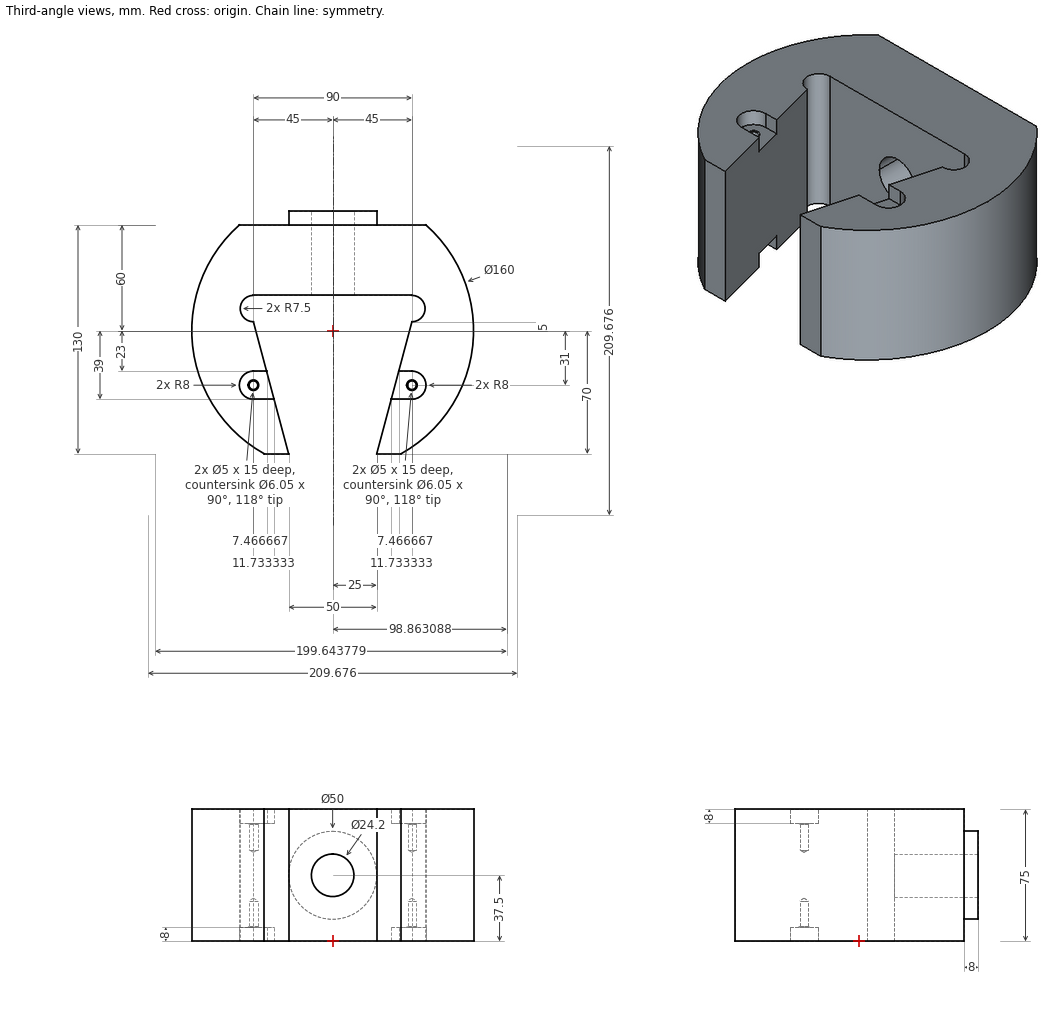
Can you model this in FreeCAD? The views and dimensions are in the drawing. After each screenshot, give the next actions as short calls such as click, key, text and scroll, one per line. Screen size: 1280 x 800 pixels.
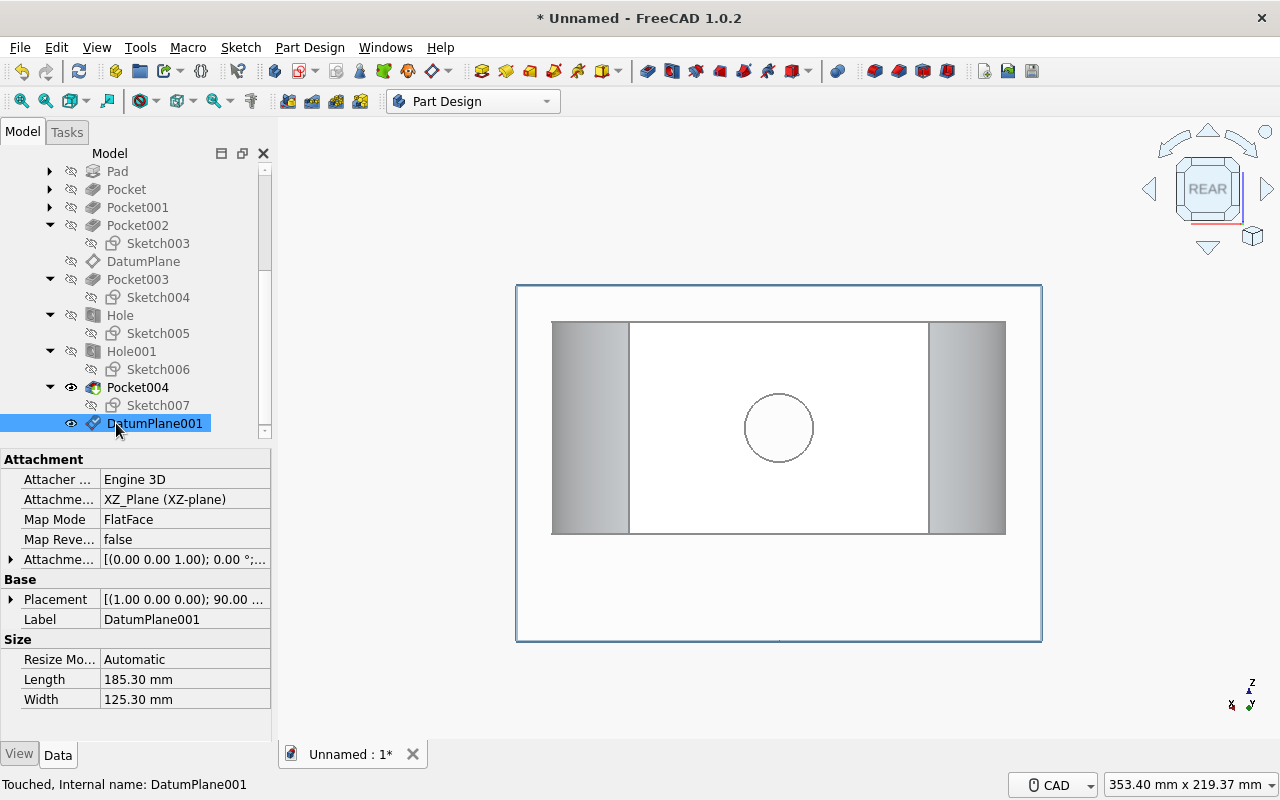
click(300, 72)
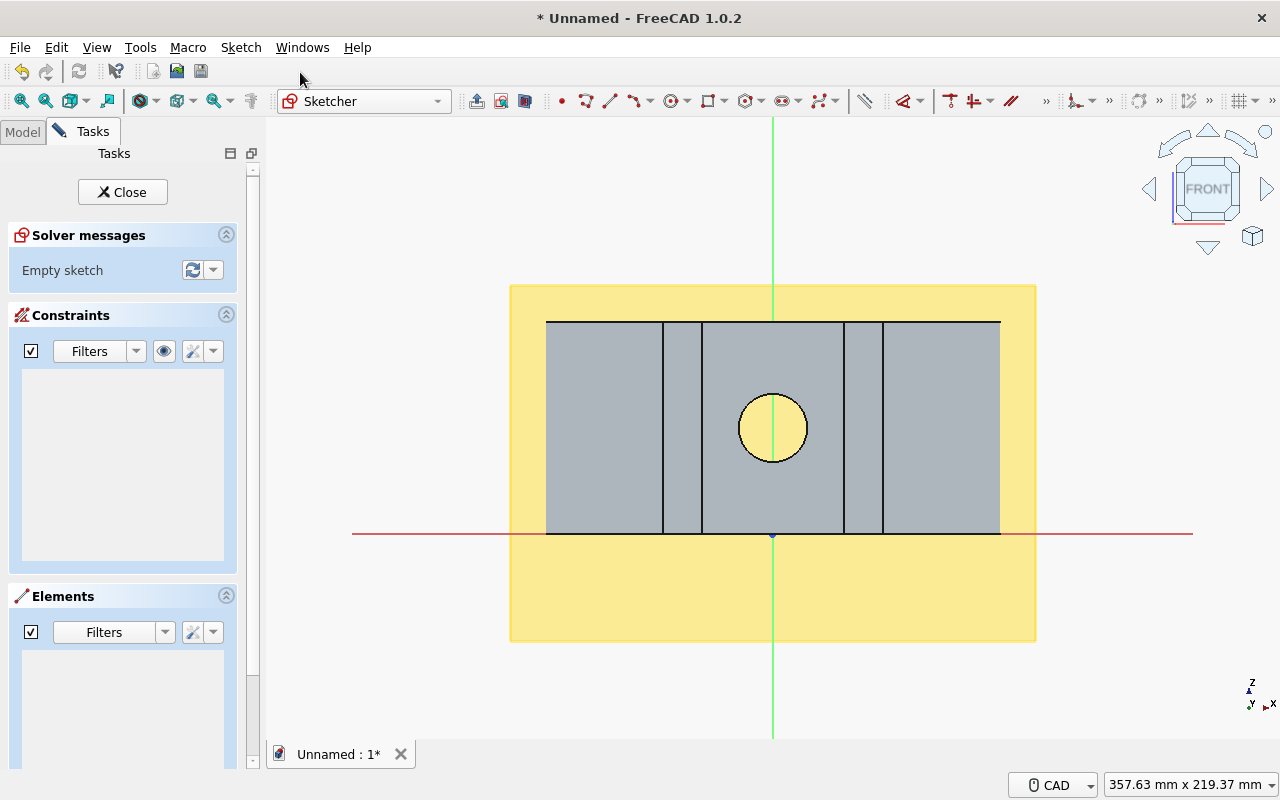
key(q)
key(s)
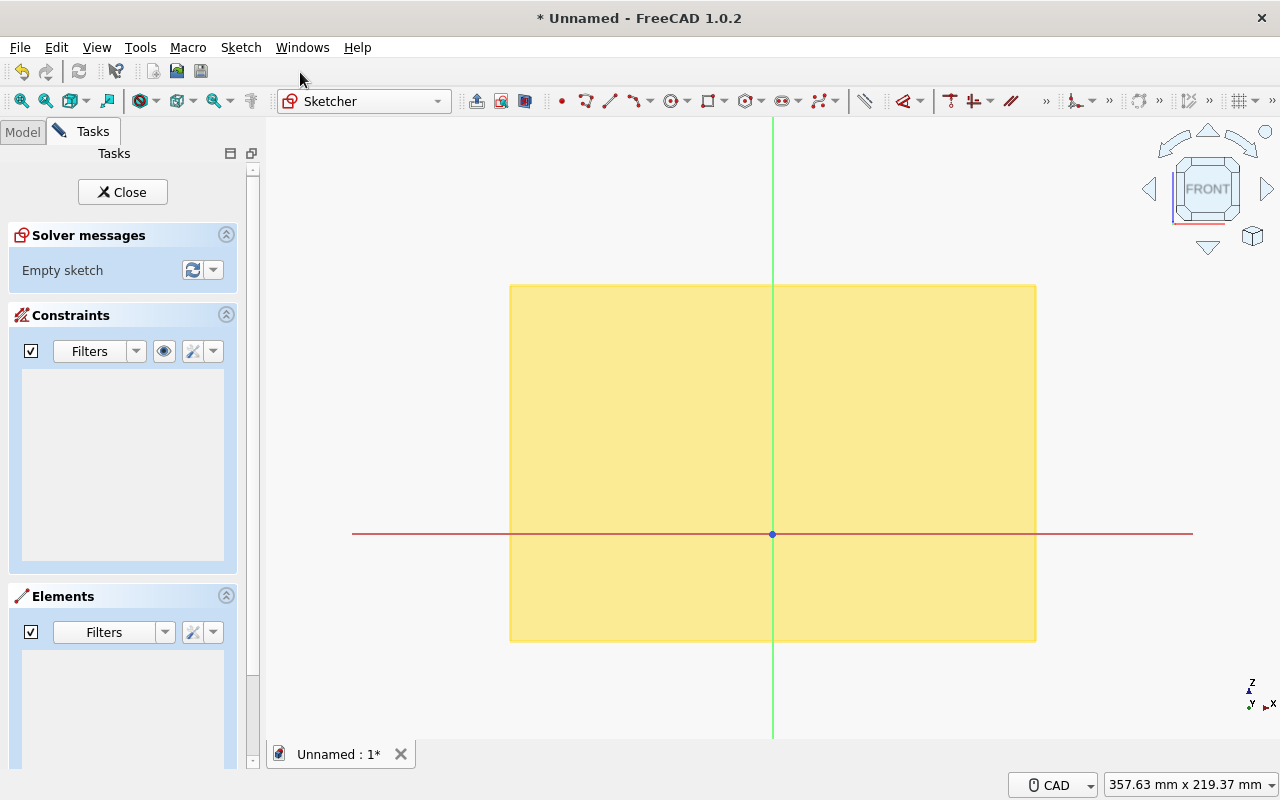
scroll(829, 460, up, 4)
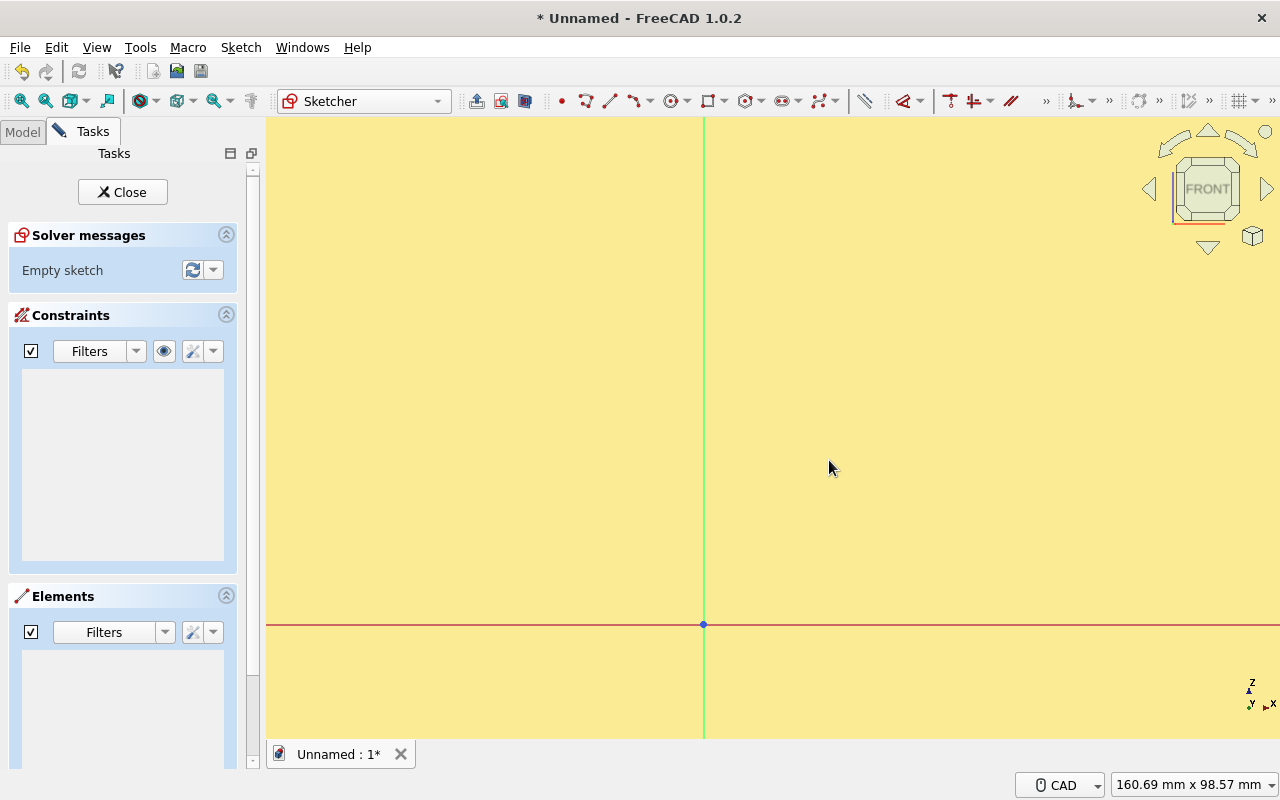
click(672, 102)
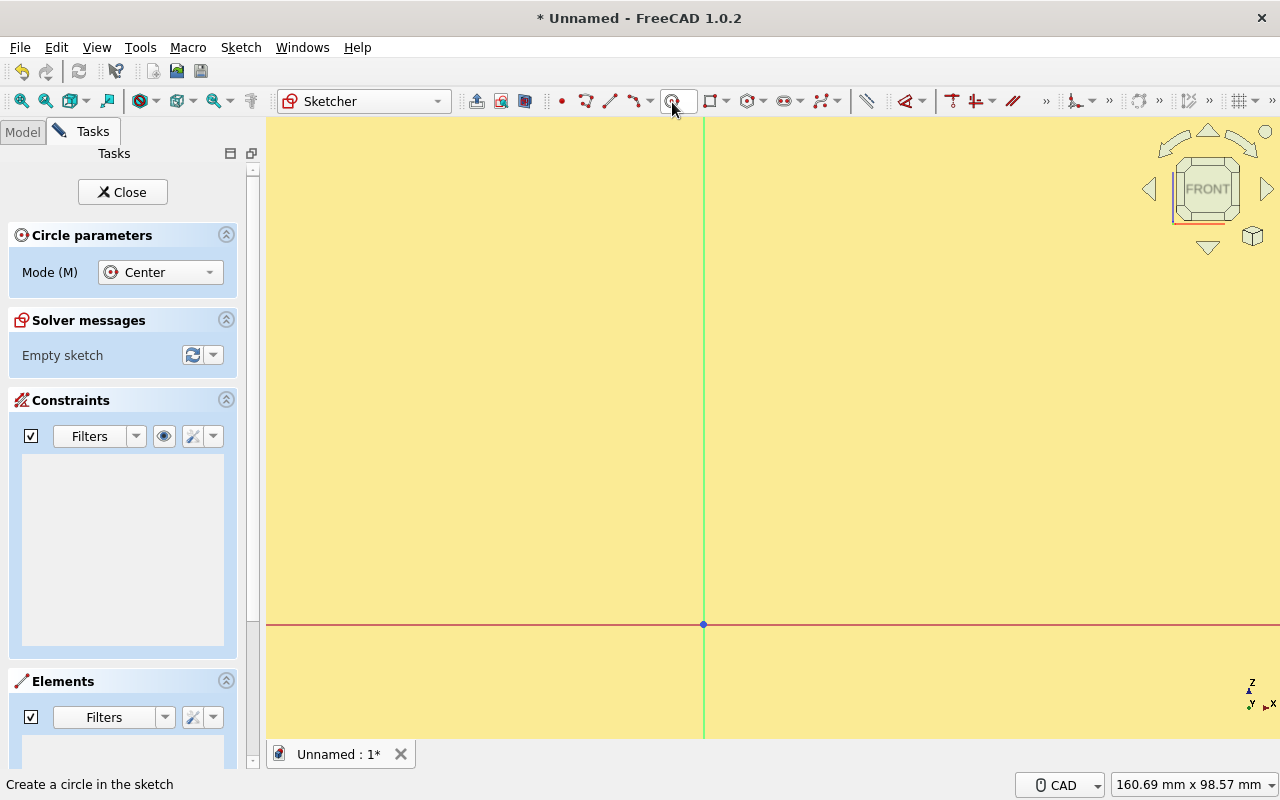
click(704, 388)
move(815, 277)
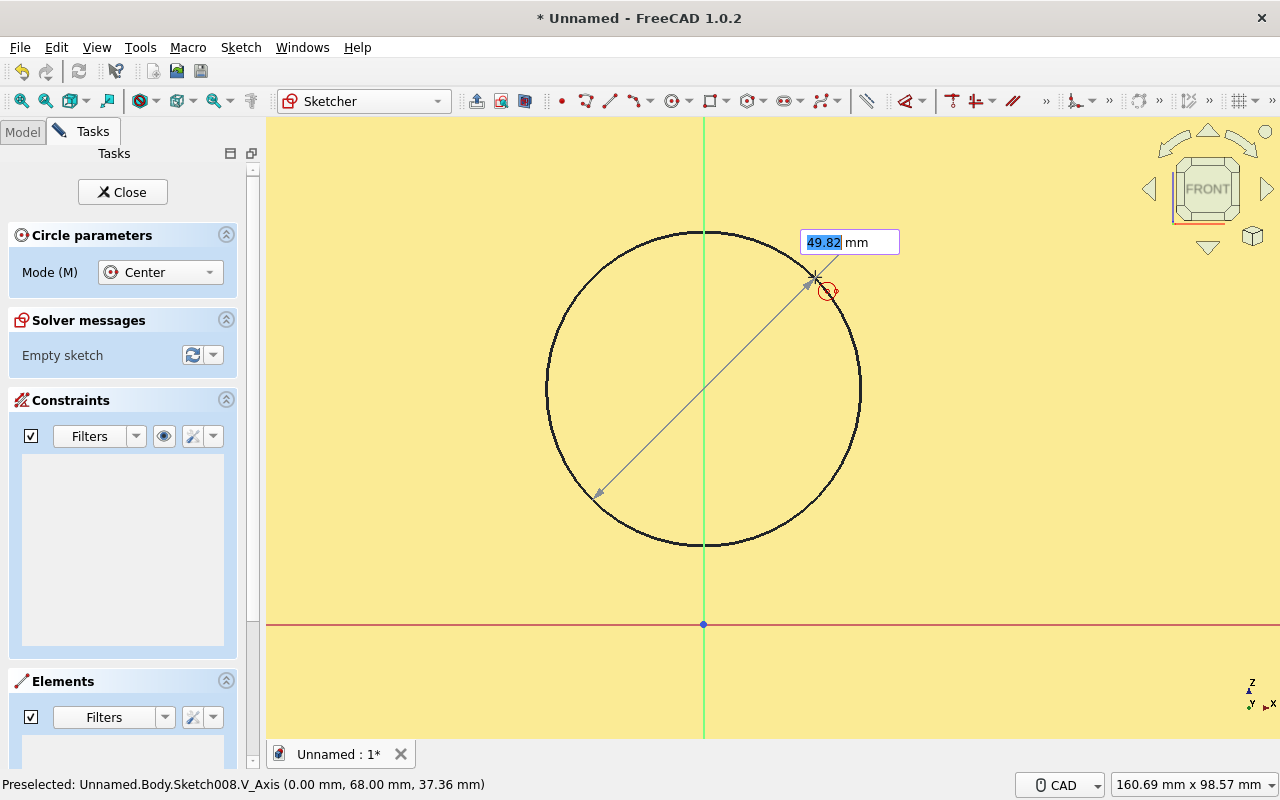
text(50)
key(Return)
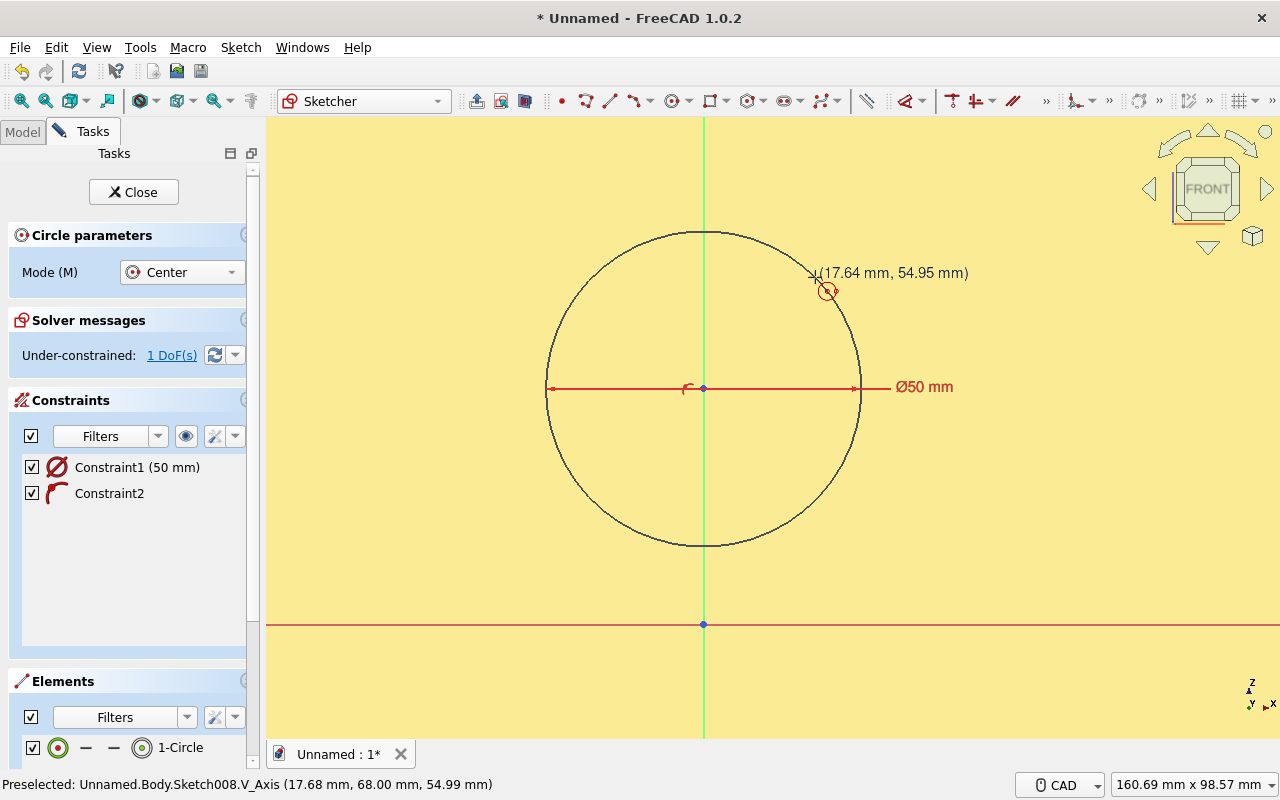
click(704, 389)
move(758, 334)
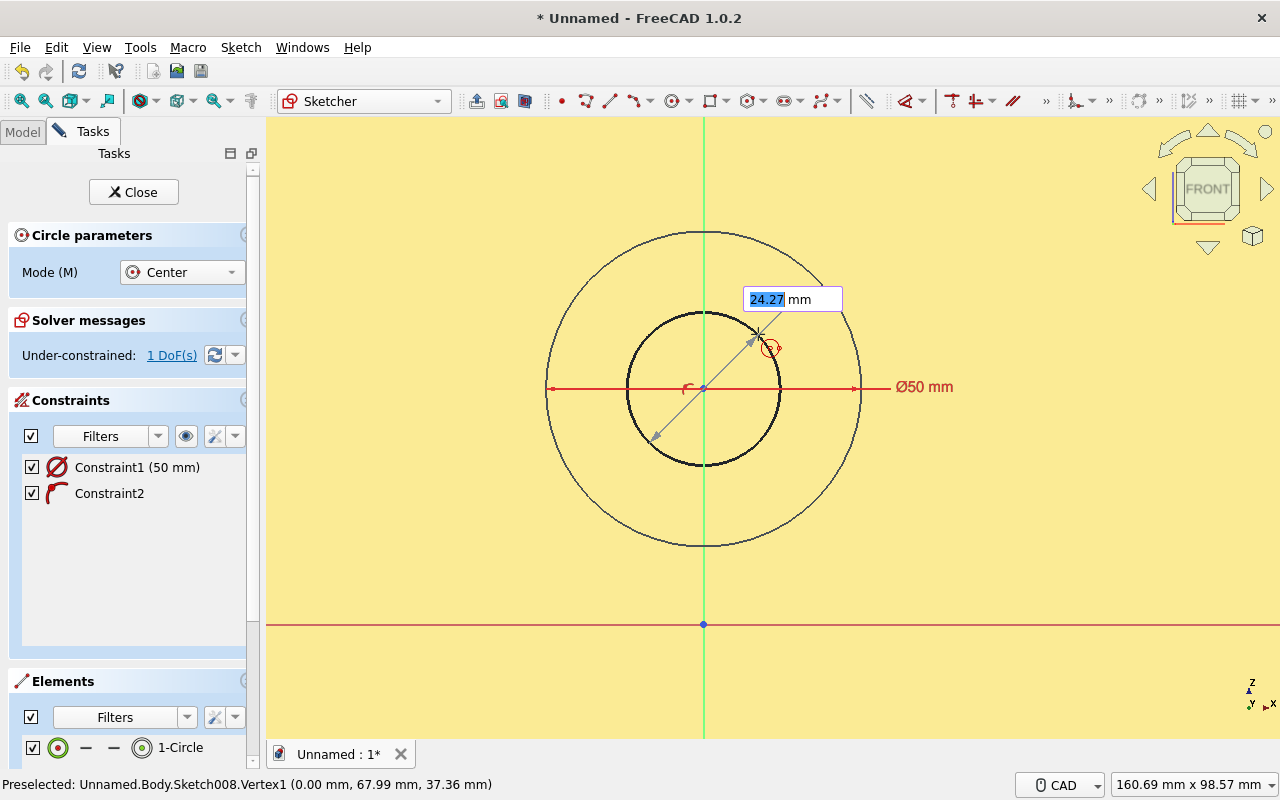
text(24.2)
key(Return)
key(Escape)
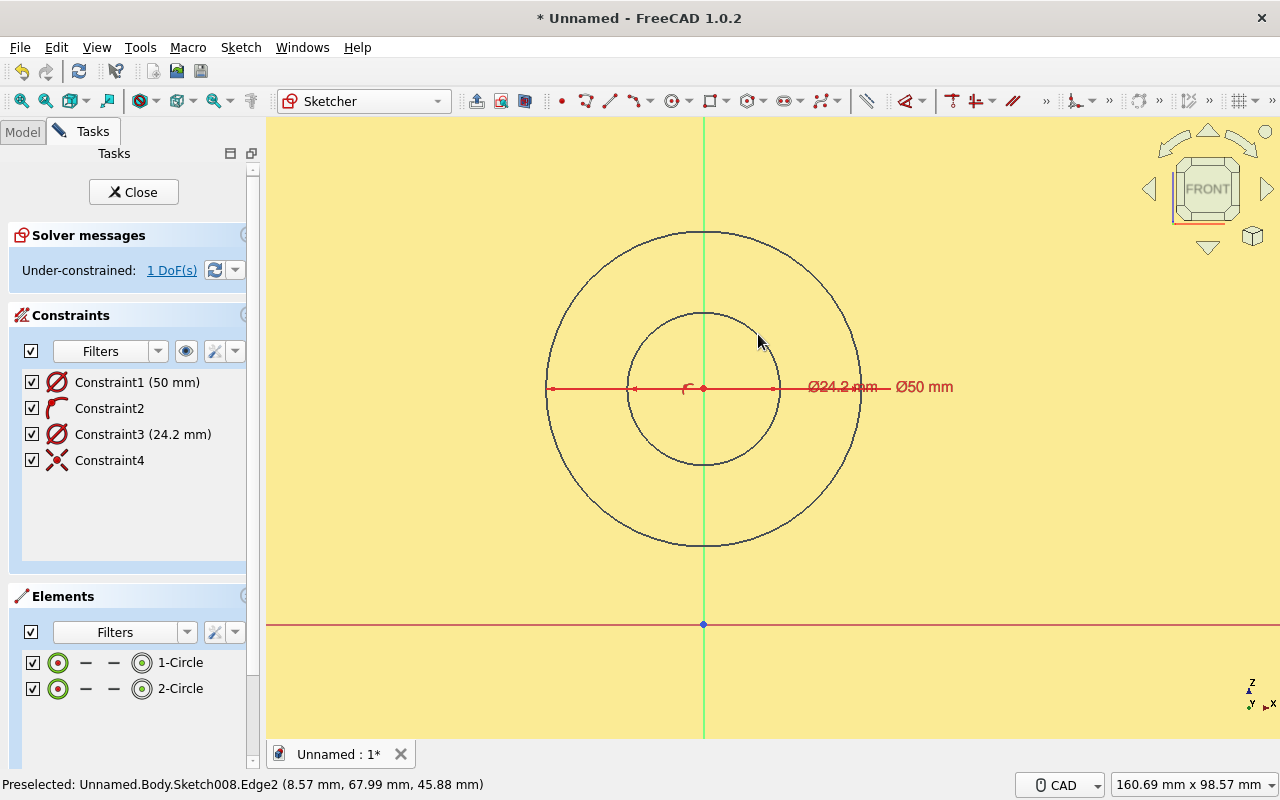
key(d)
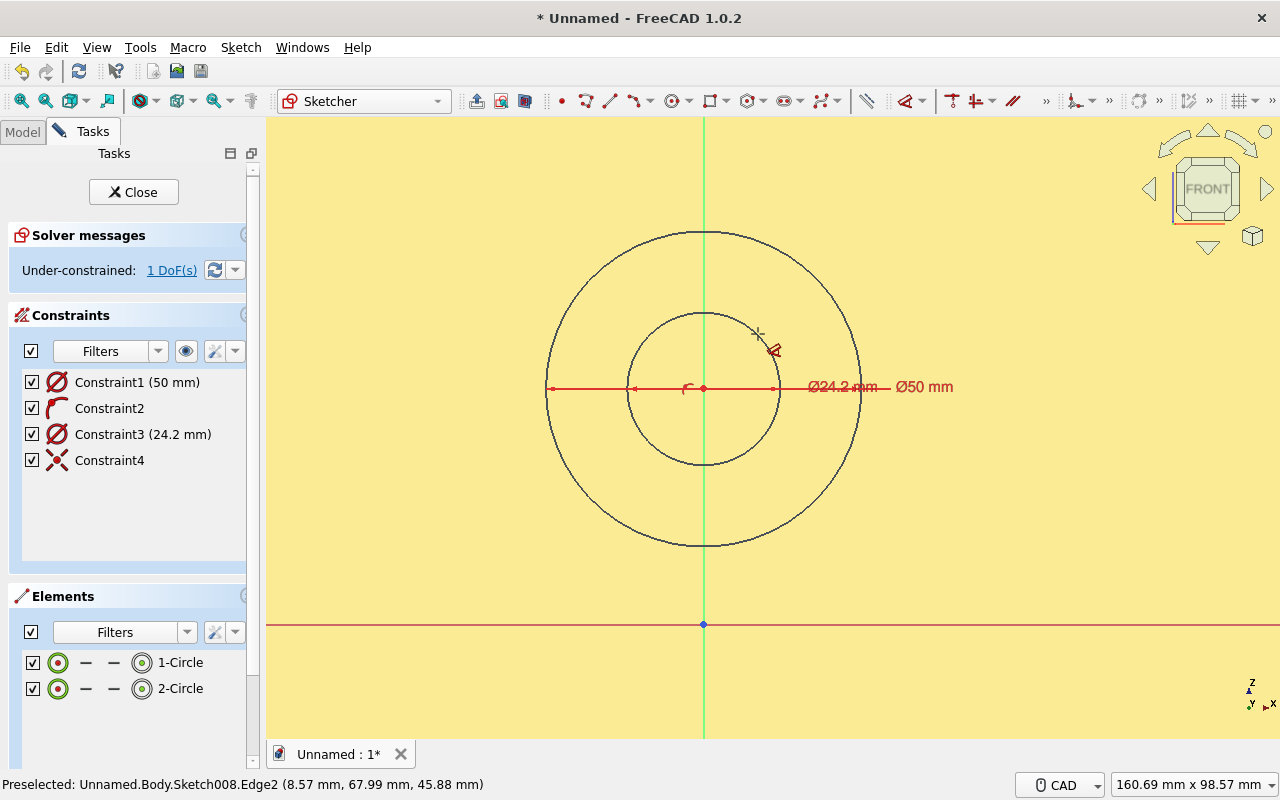
click(704, 389)
click(738, 507)